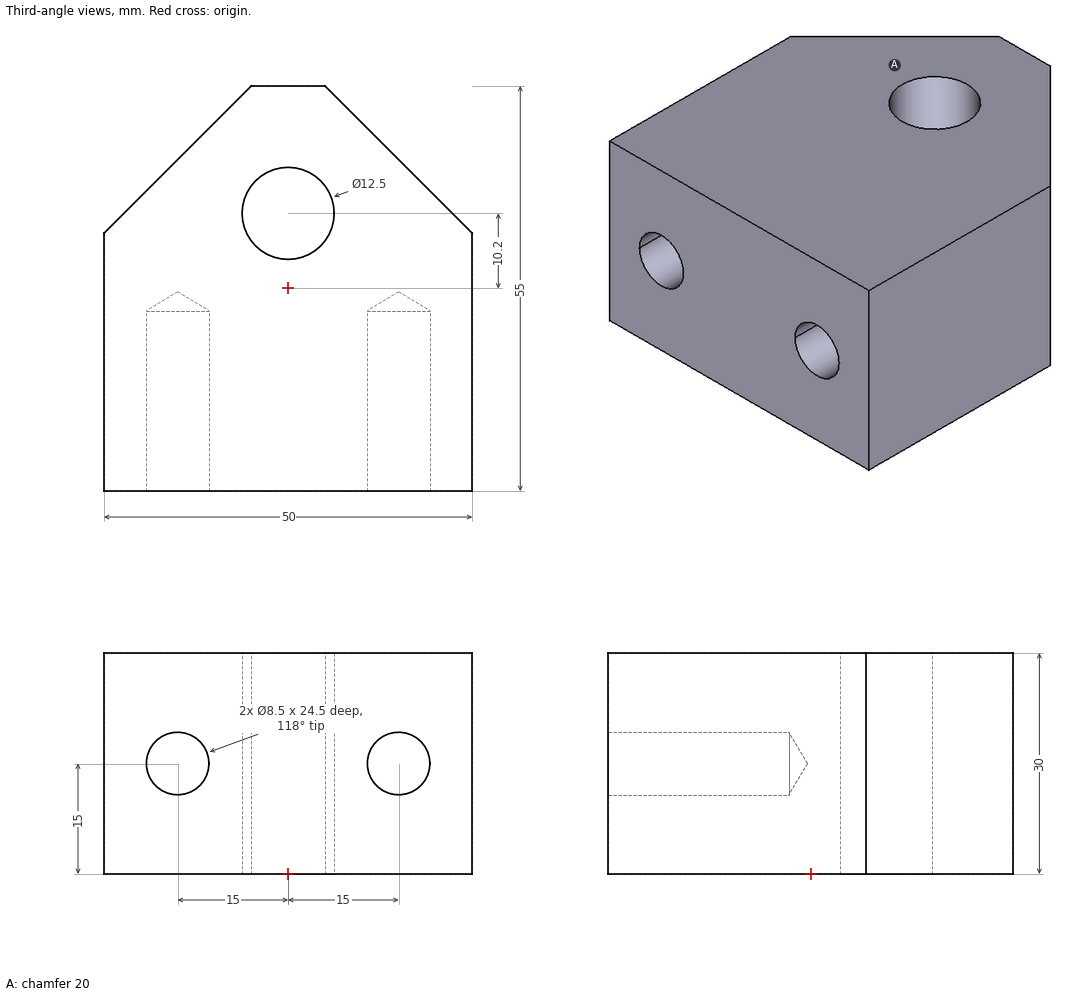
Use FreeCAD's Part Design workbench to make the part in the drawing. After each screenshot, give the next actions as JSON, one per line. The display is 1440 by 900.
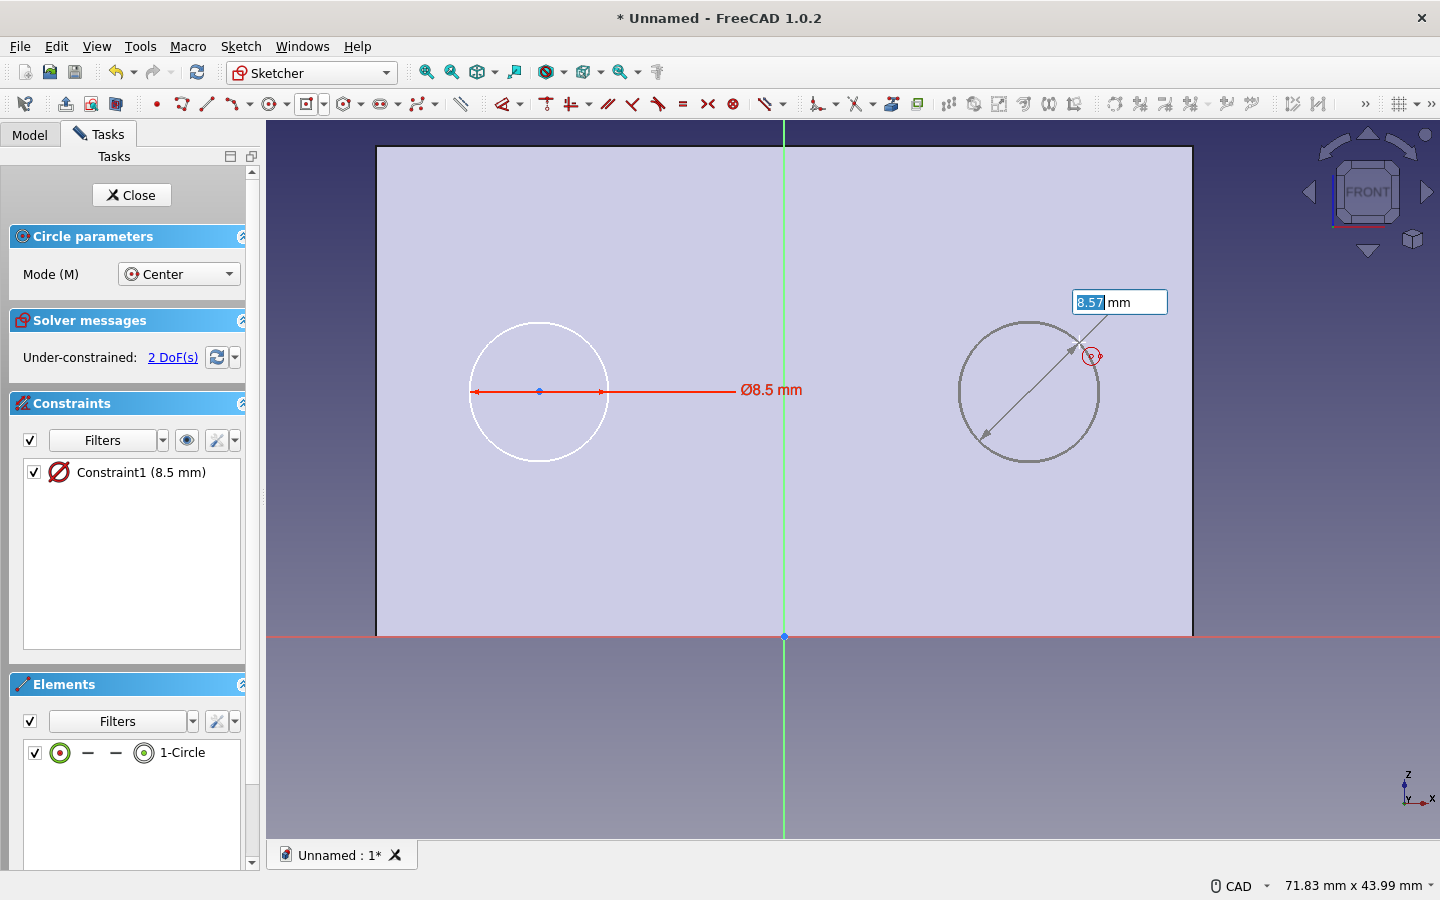
{"action": "type", "text": "8.5"}
{"action": "key", "text": "Return"}
{"action": "key", "text": "Escape"}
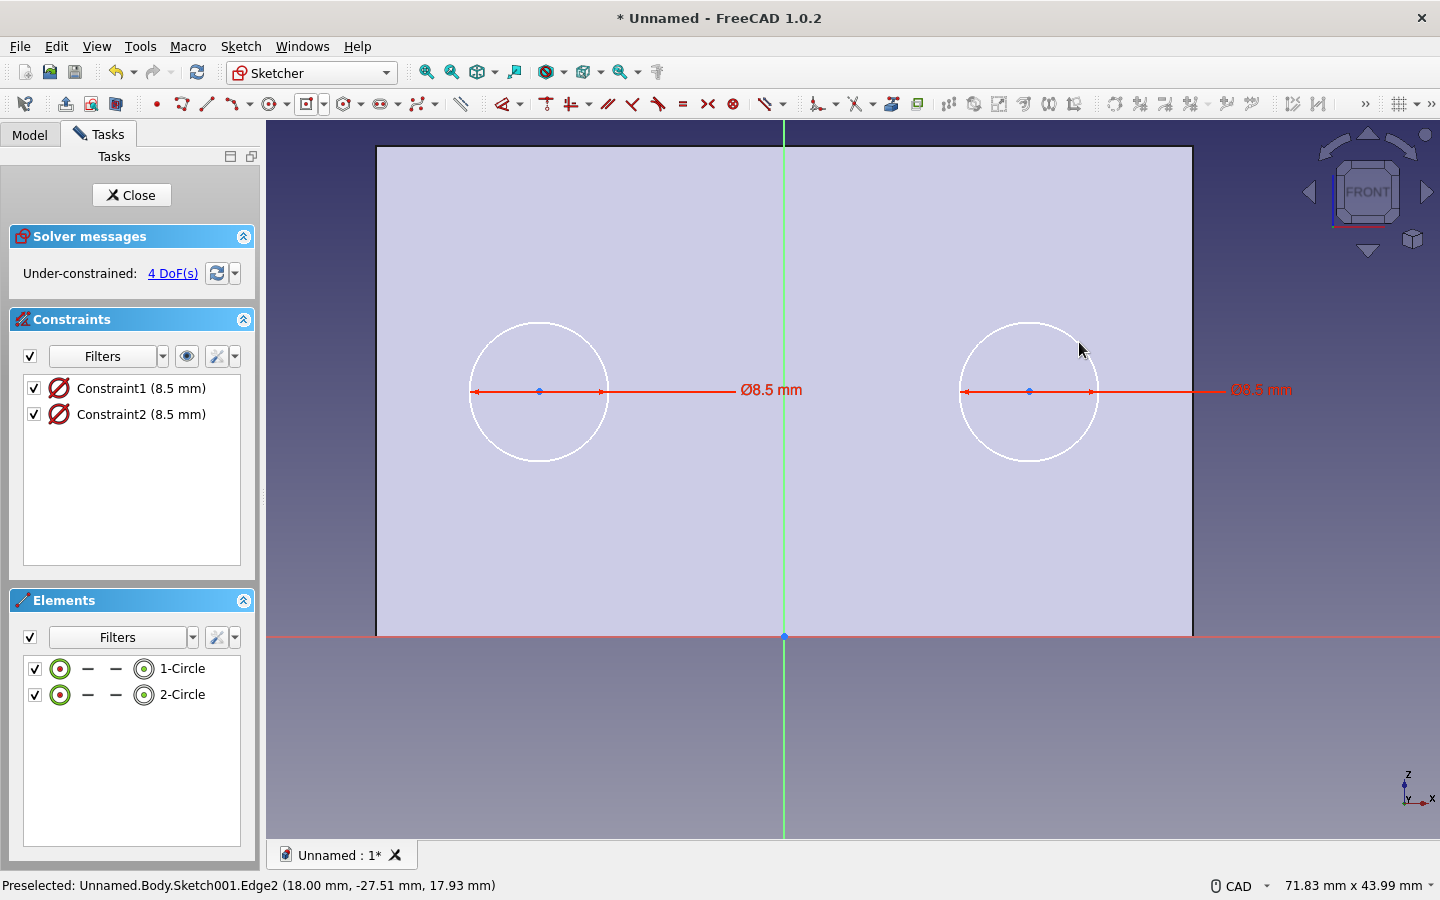
{"action": "left_click", "coordinate": [539, 392]}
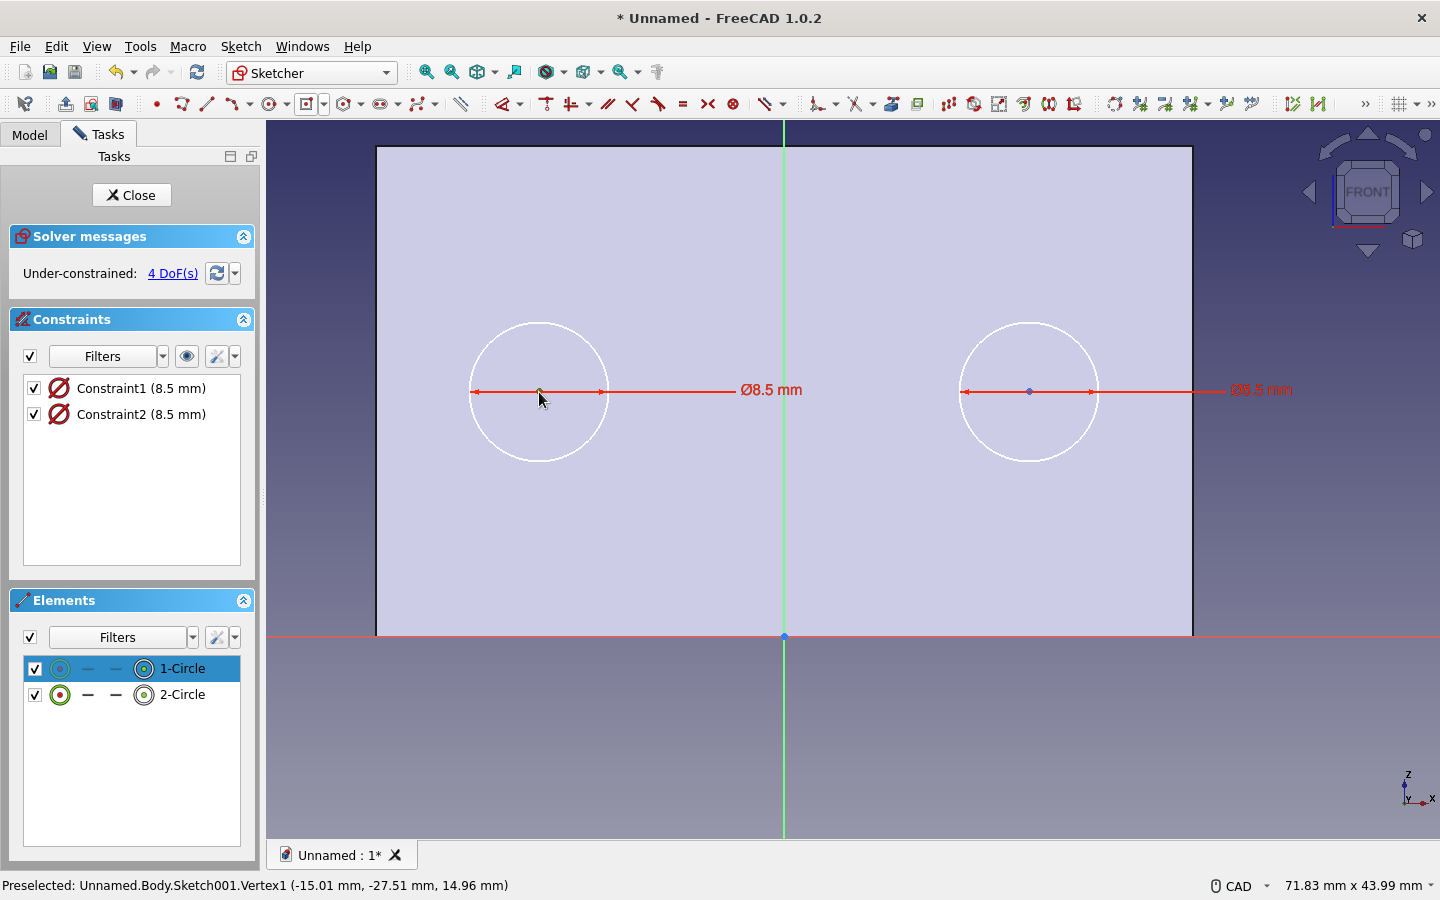
{"action": "left_click", "coordinate": [1029, 392]}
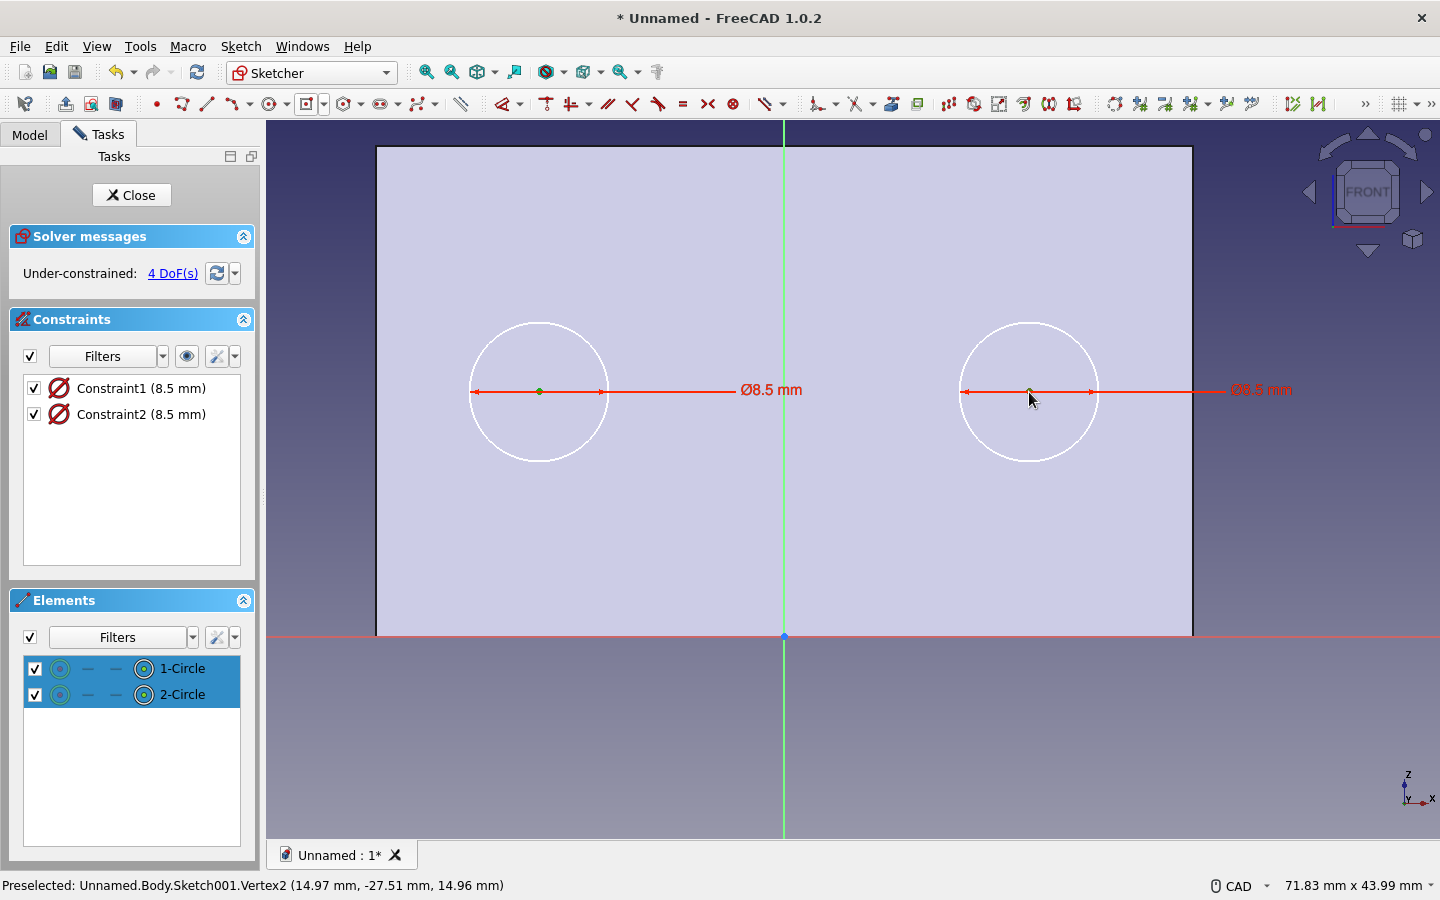
{"action": "key", "text": "h"}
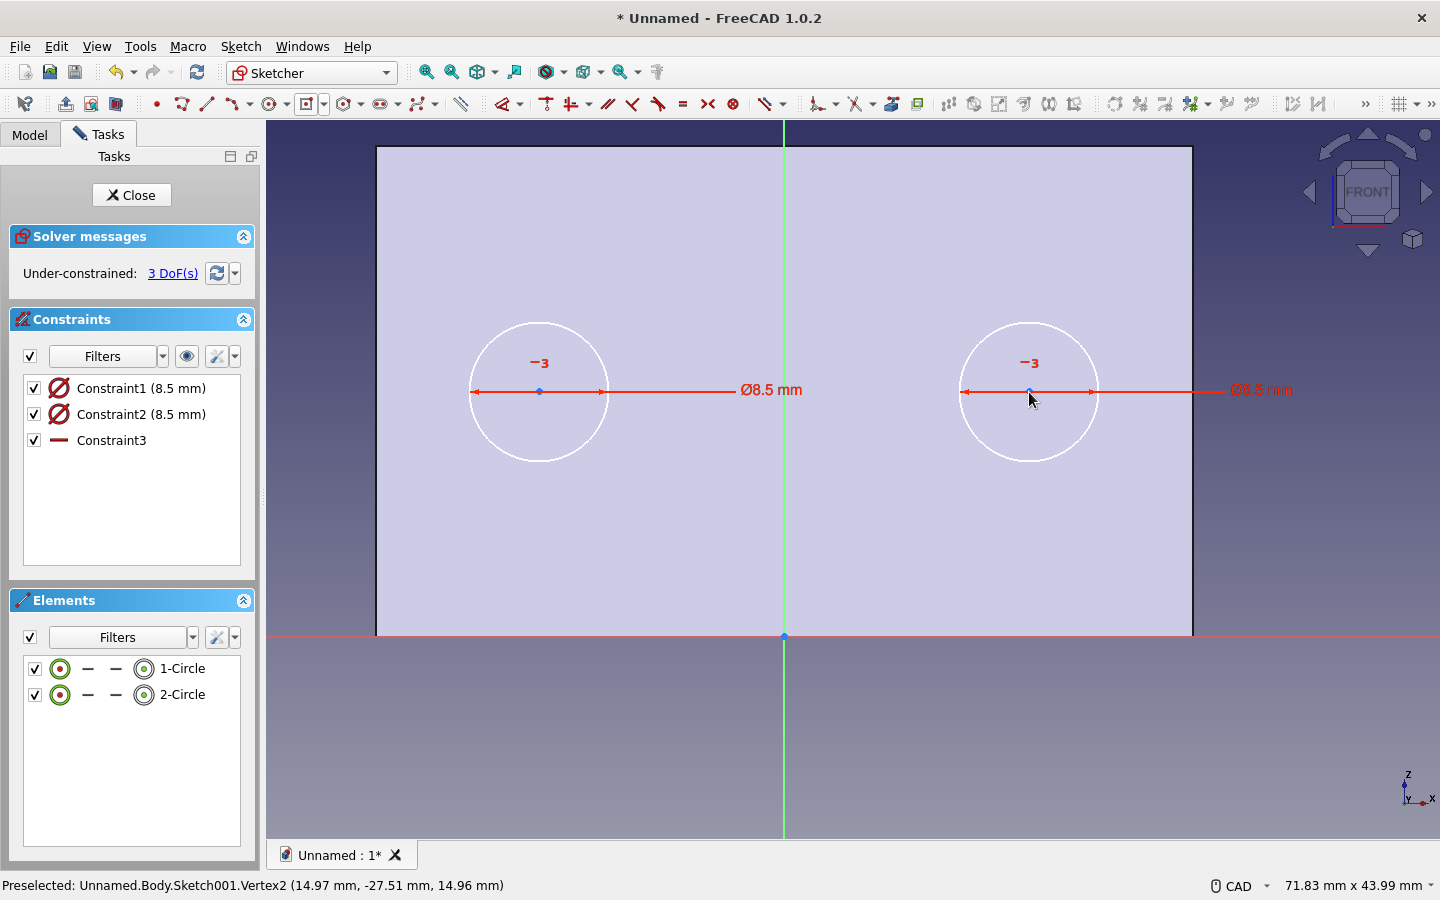
{"action": "key", "text": "d"}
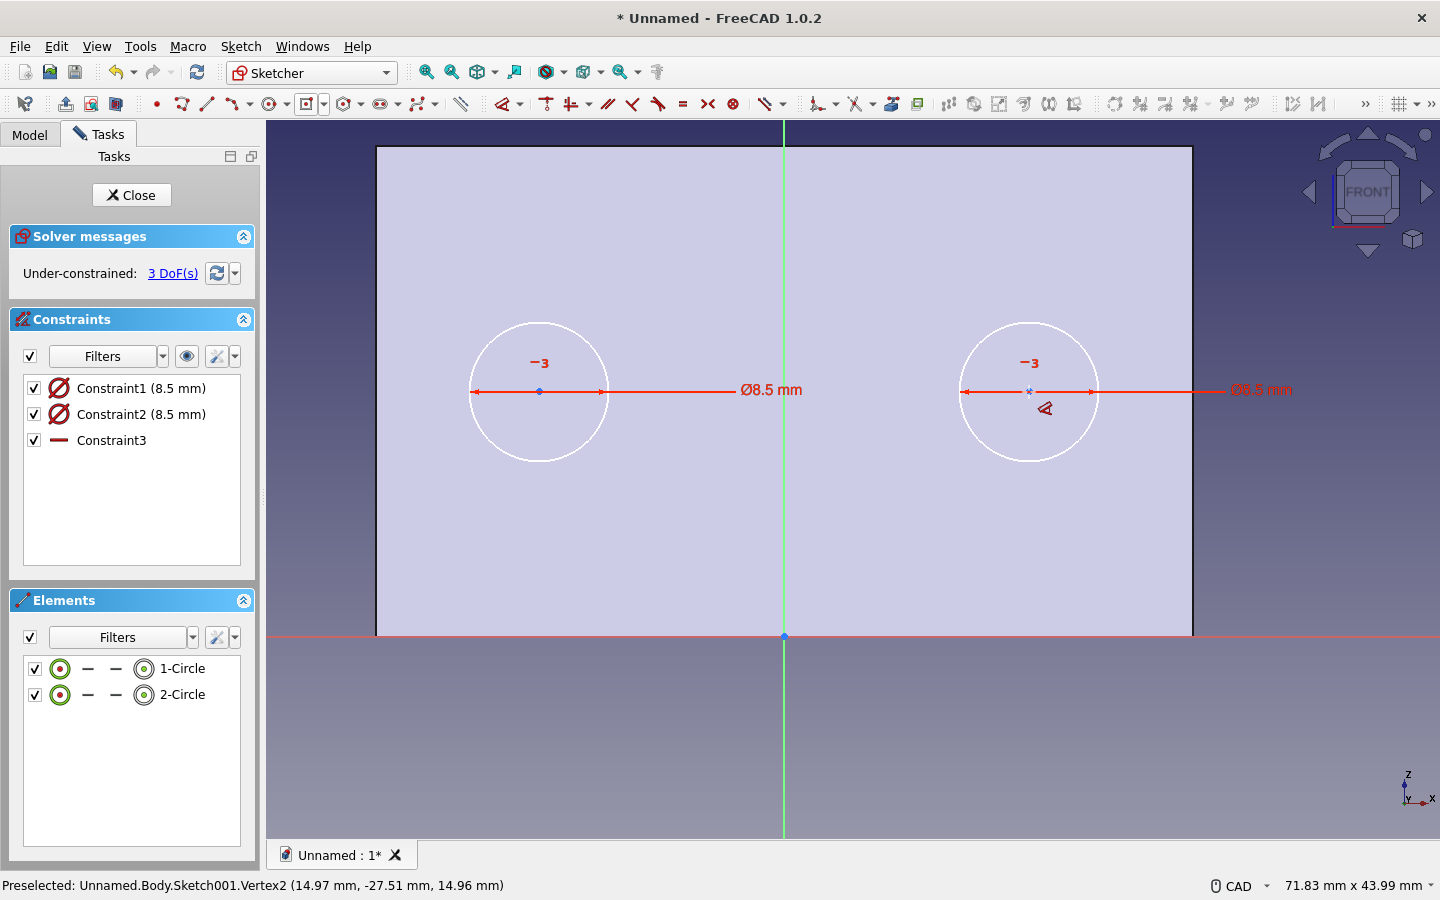
{"action": "left_click", "coordinate": [539, 392]}
{"action": "left_click", "coordinate": [662, 671]}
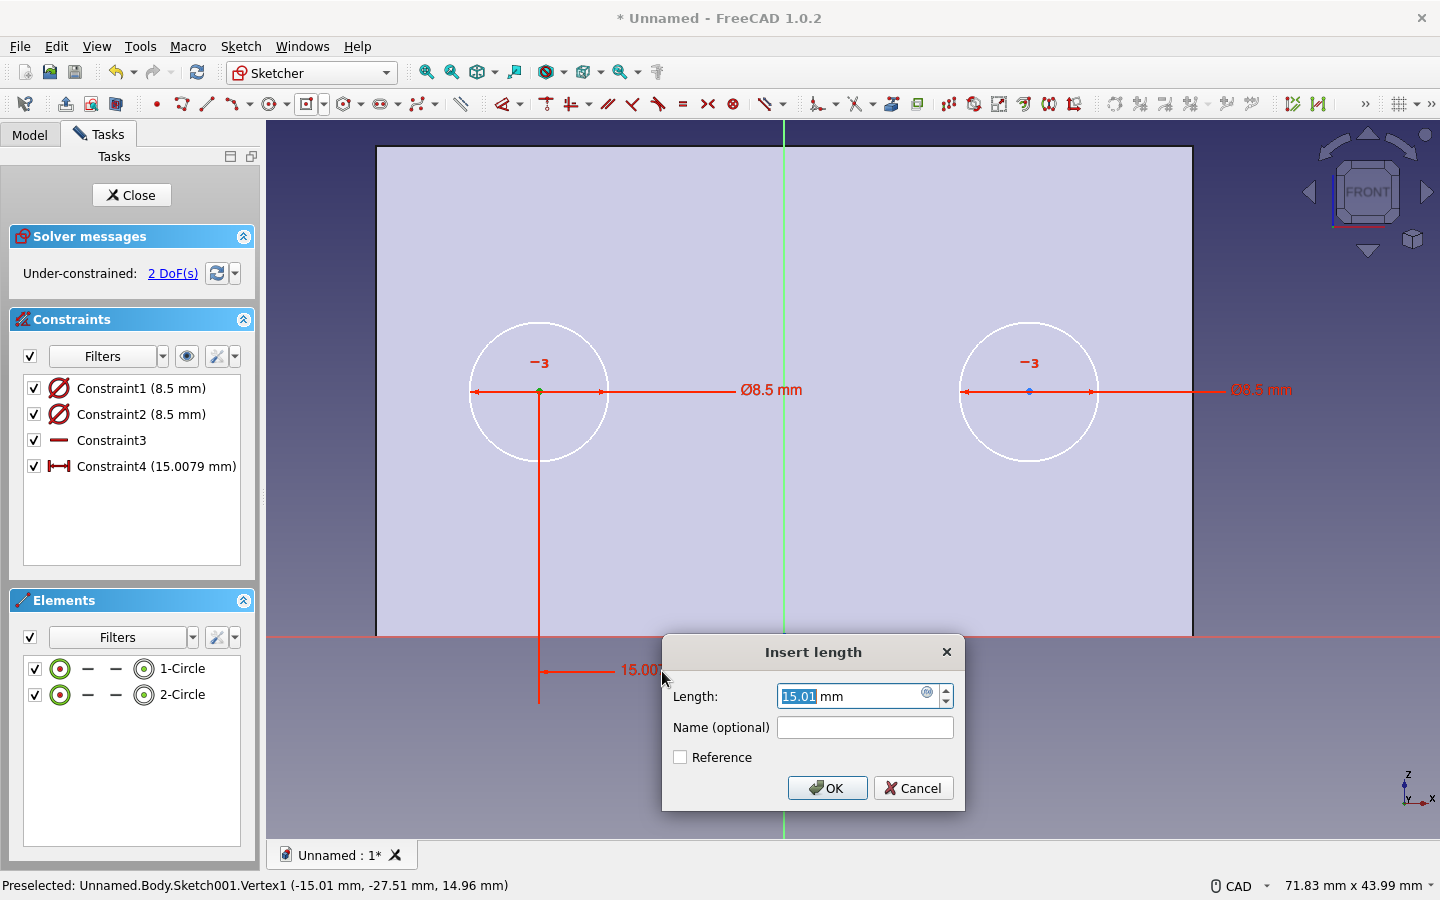
{"action": "type", "text": "15"}
{"action": "key", "text": "Return"}